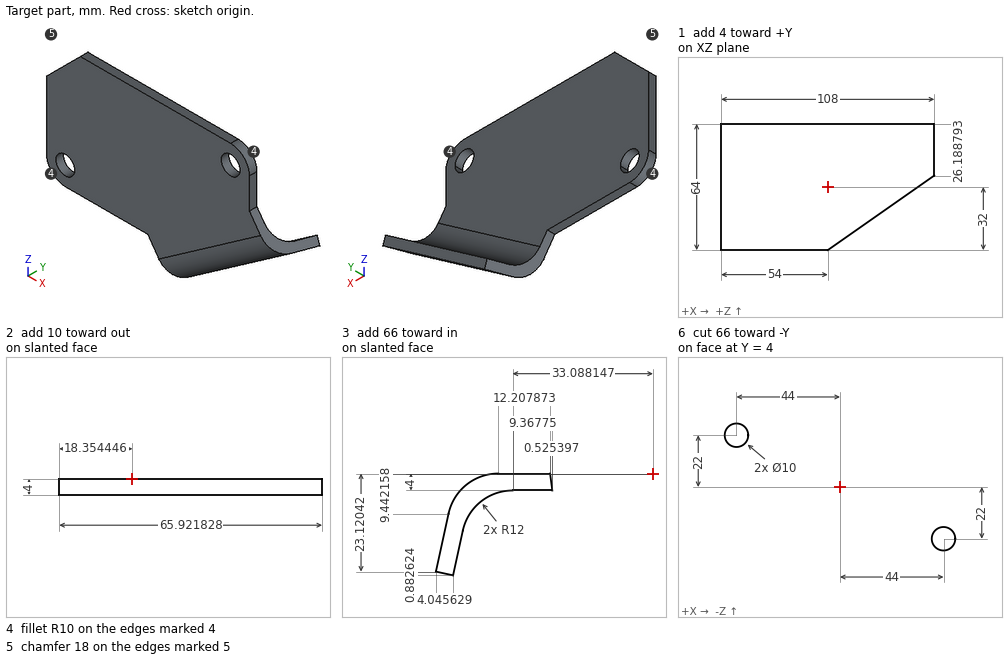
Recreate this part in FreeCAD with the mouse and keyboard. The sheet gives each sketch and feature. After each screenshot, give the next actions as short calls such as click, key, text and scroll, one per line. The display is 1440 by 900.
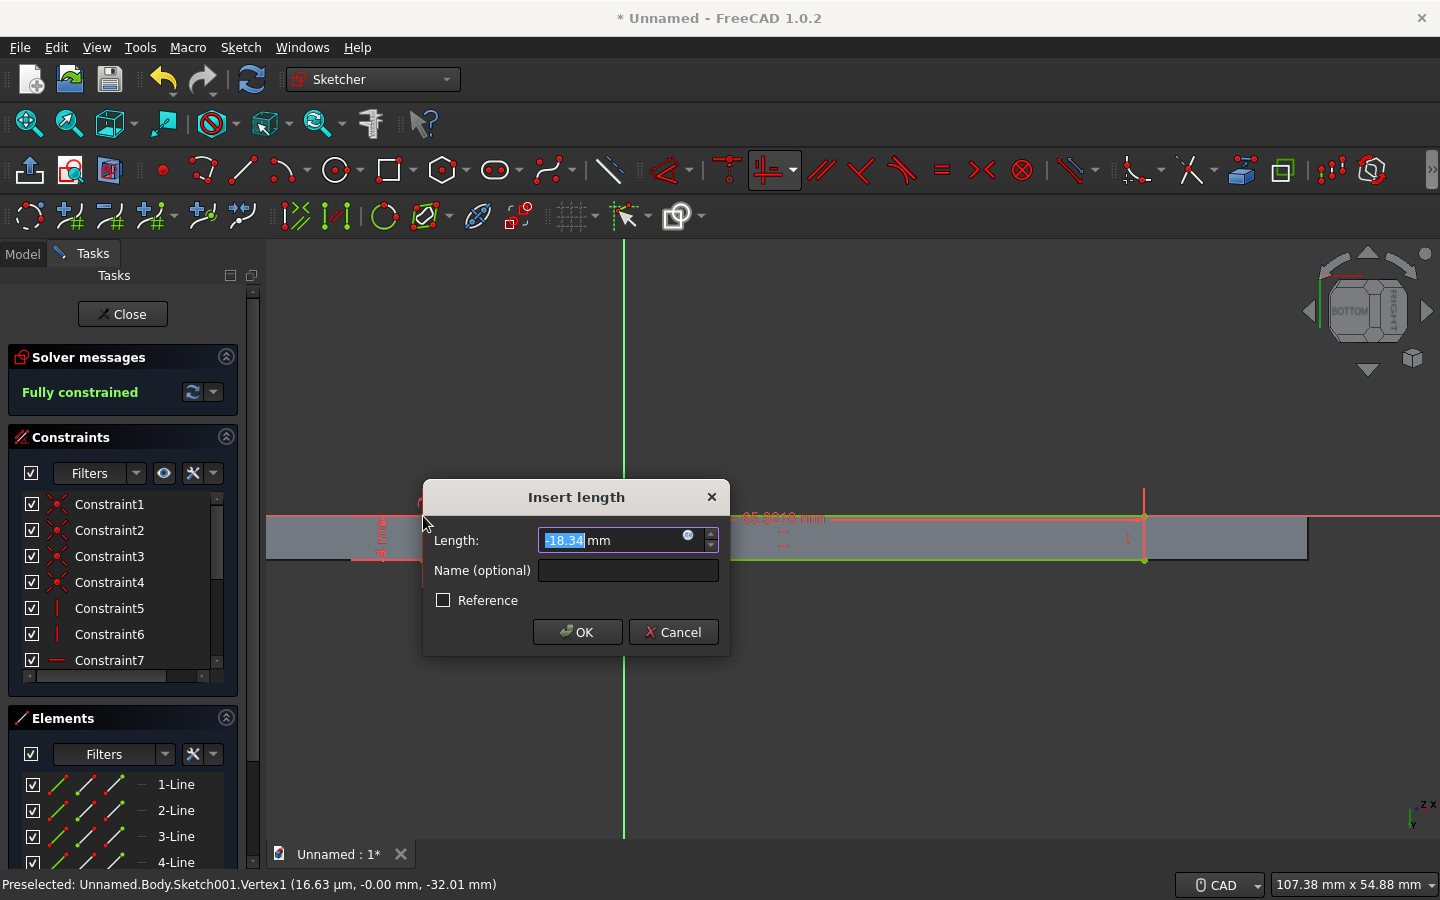
text(-18.354446)
key(Return)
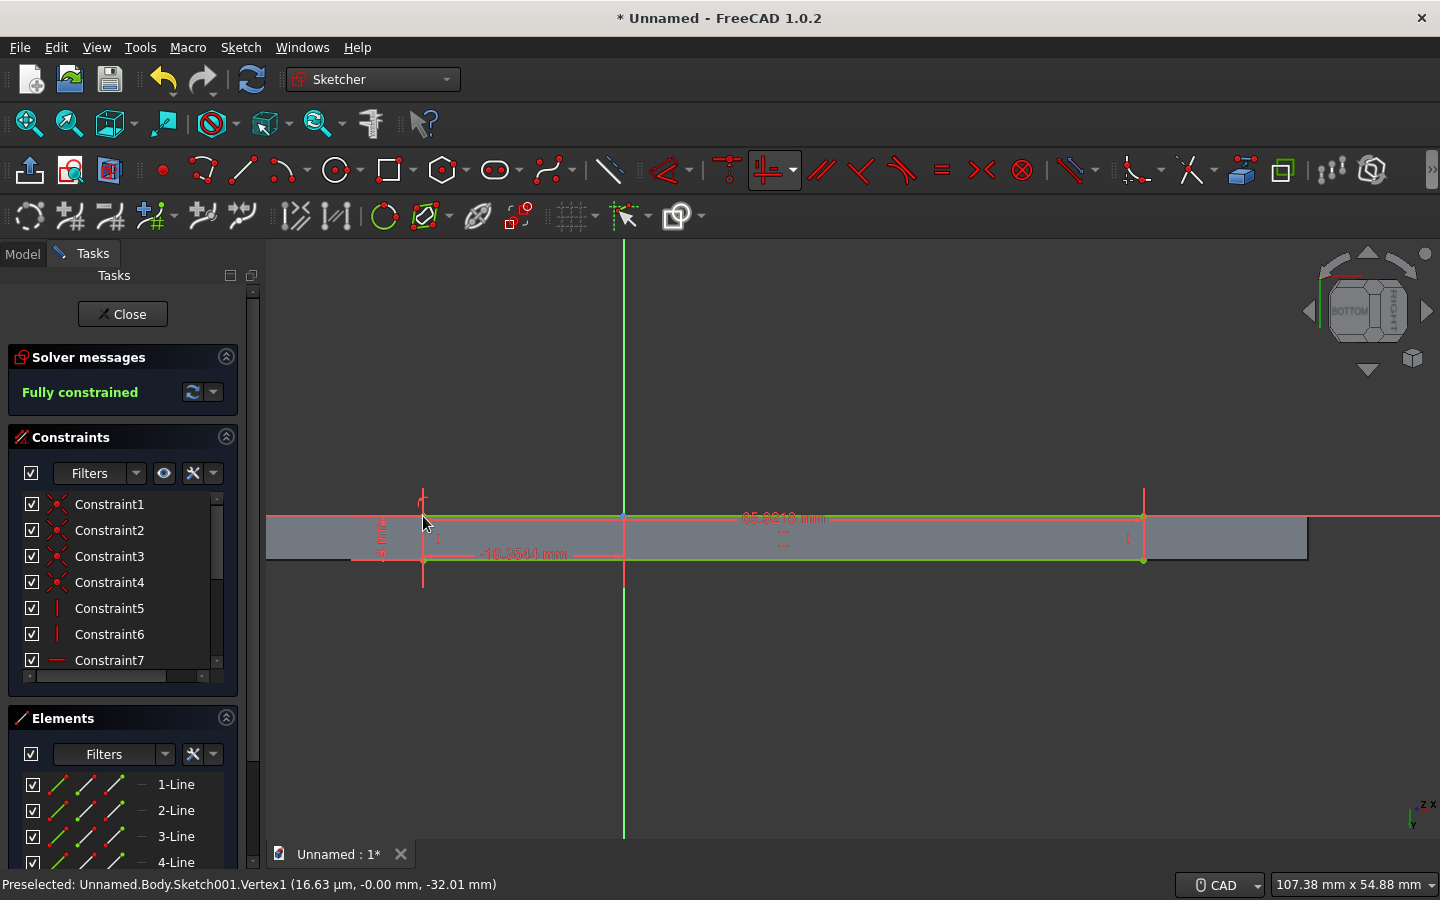
click(123, 314)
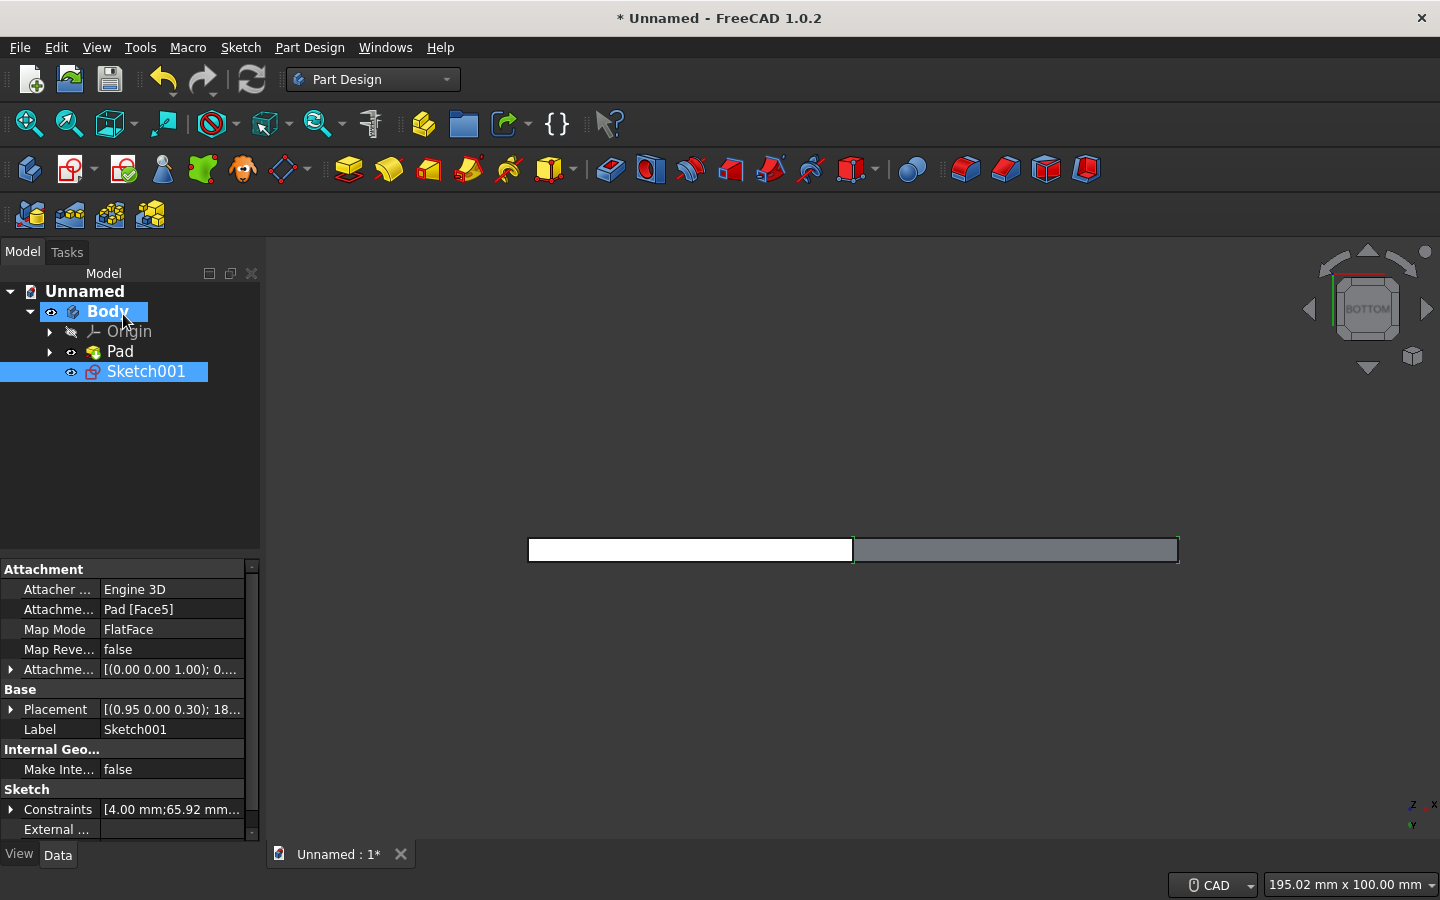
click(350, 170)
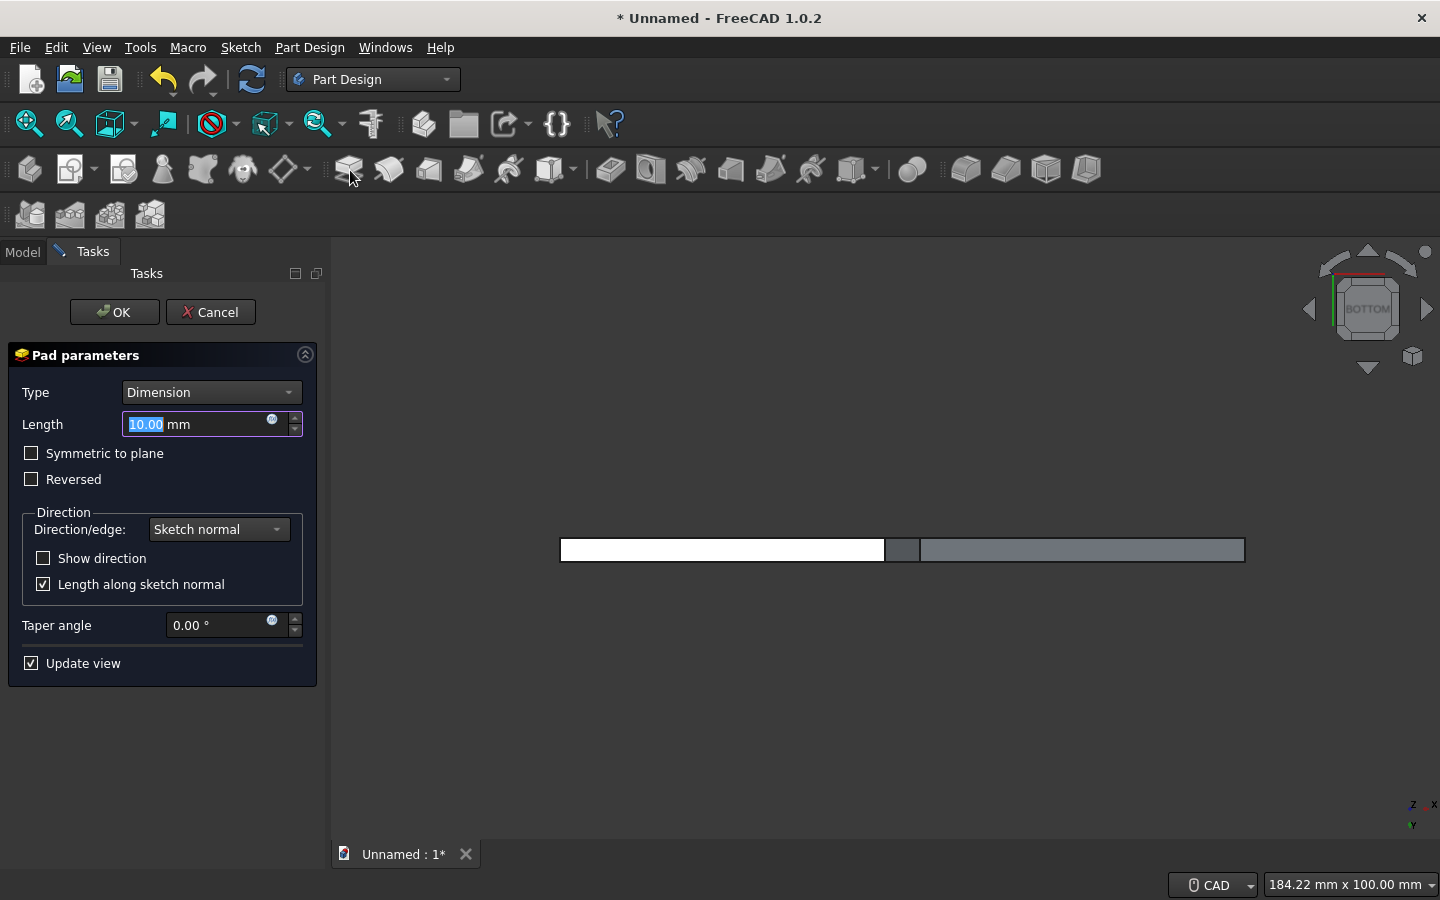
text(10)
key(Tab)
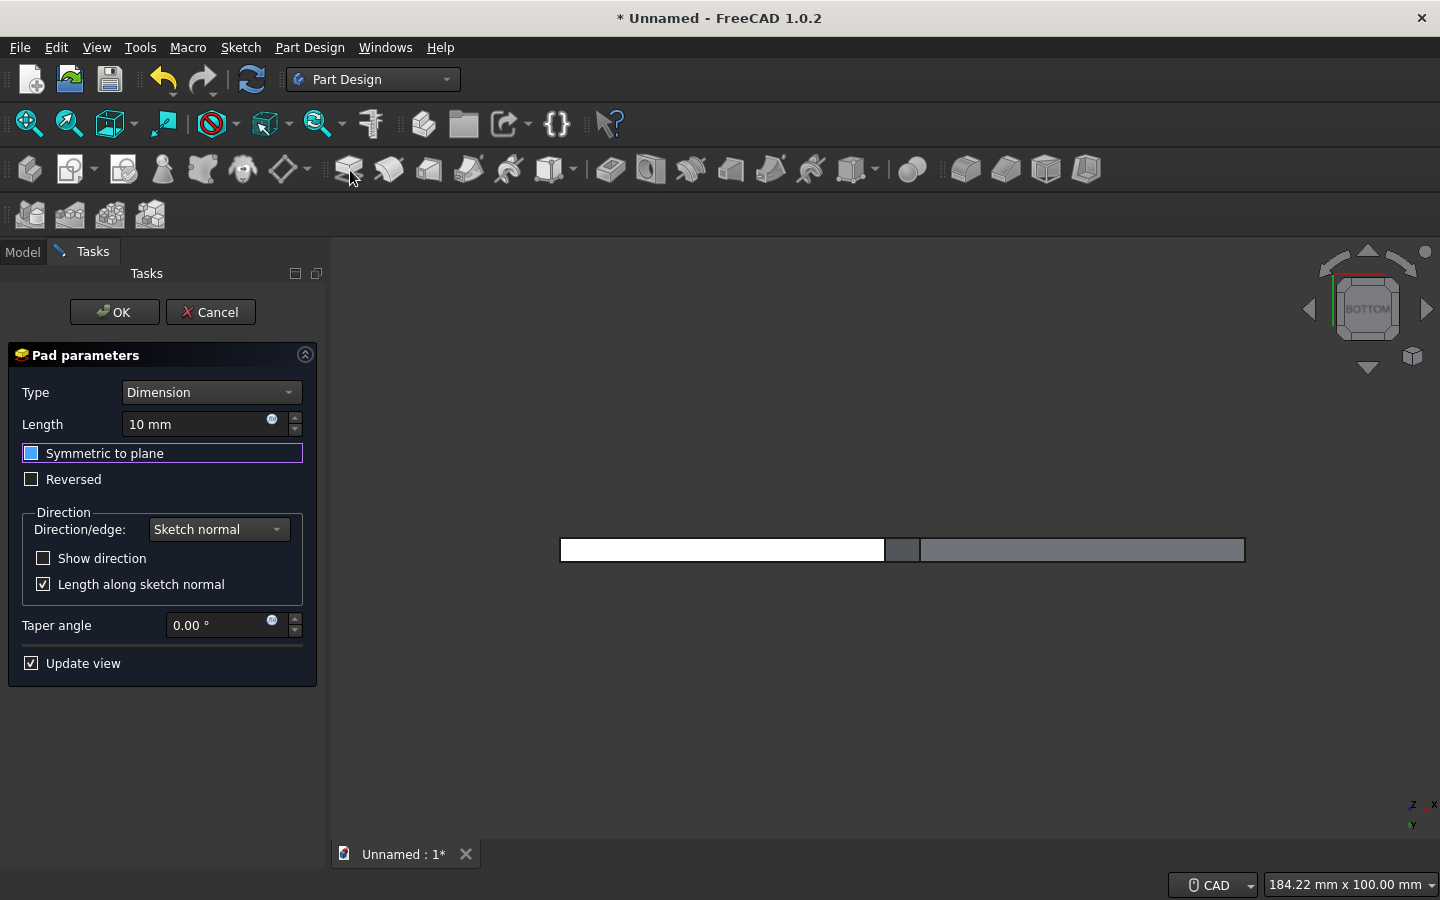
click(115, 312)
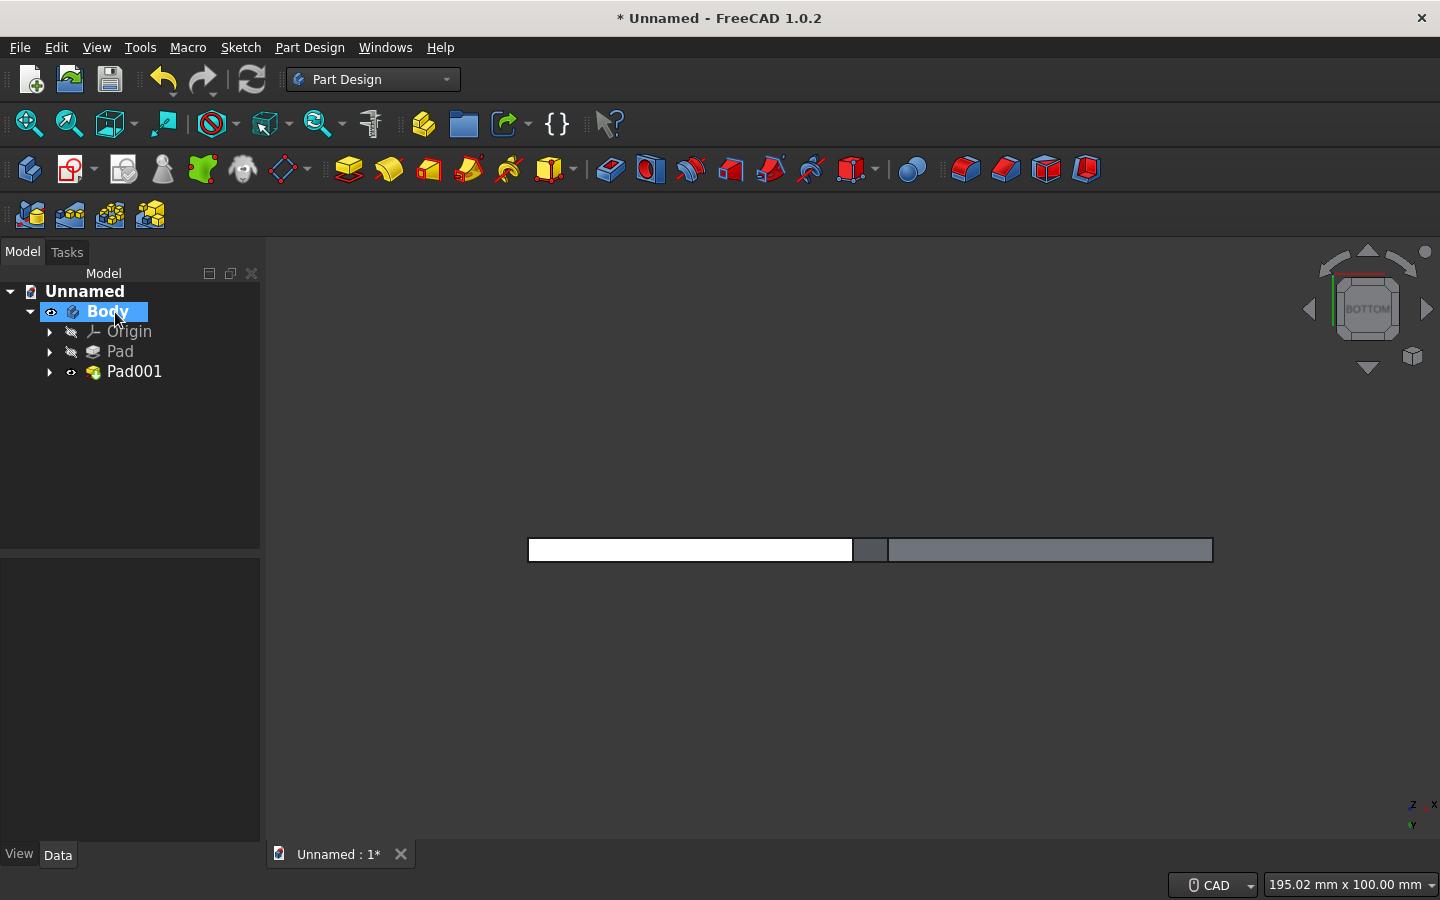
key(0)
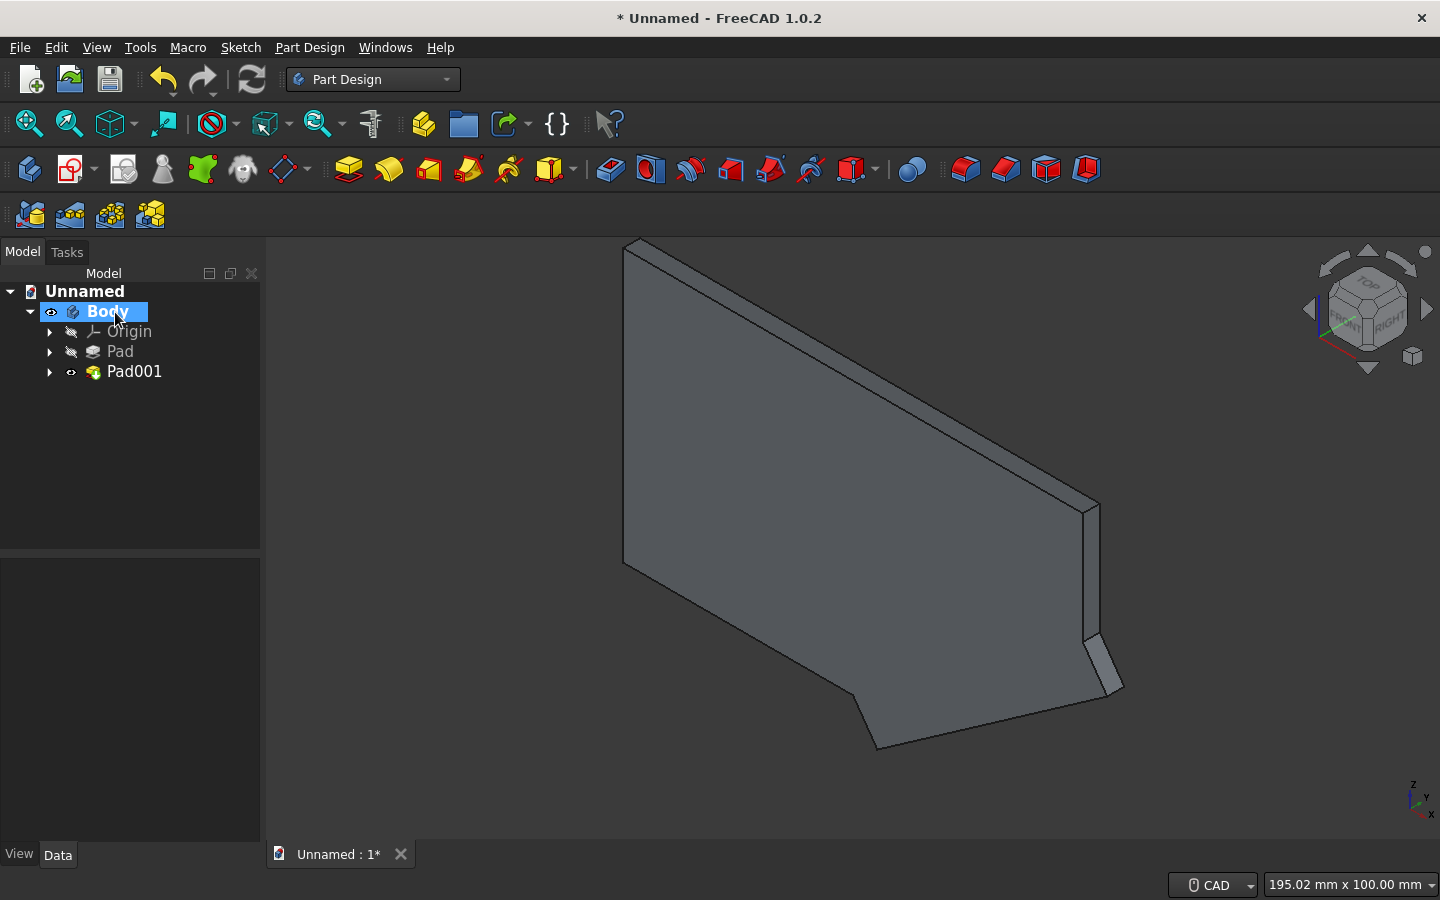
key(v)
key(f)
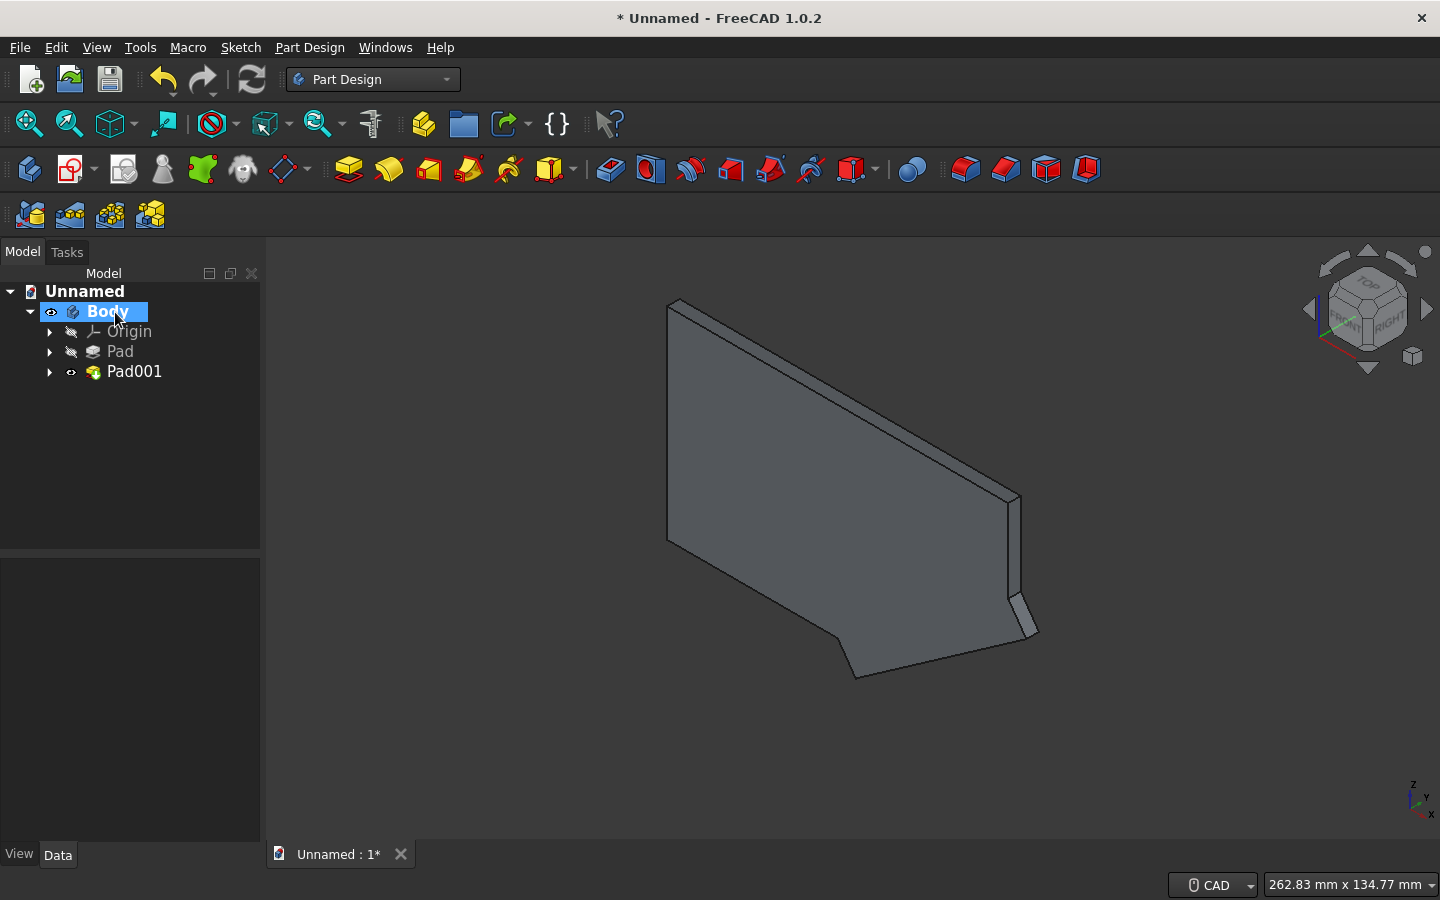
key(3)